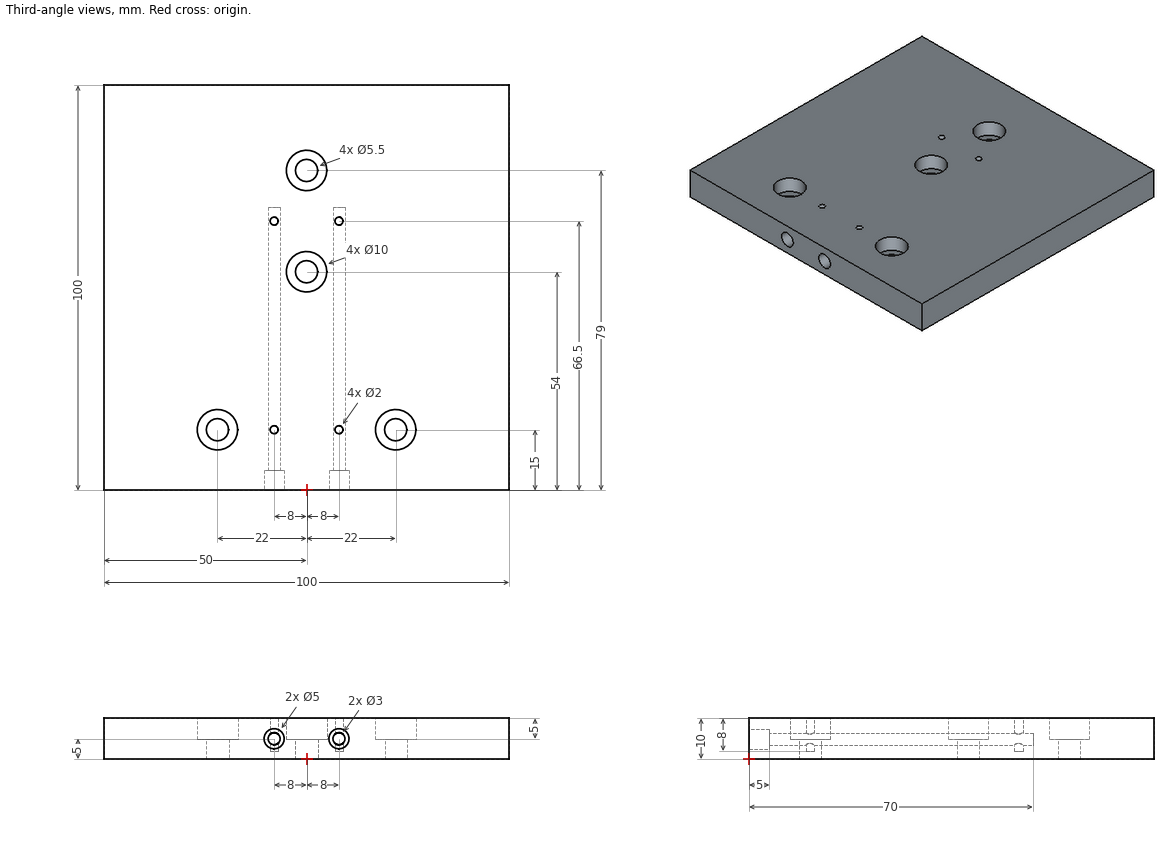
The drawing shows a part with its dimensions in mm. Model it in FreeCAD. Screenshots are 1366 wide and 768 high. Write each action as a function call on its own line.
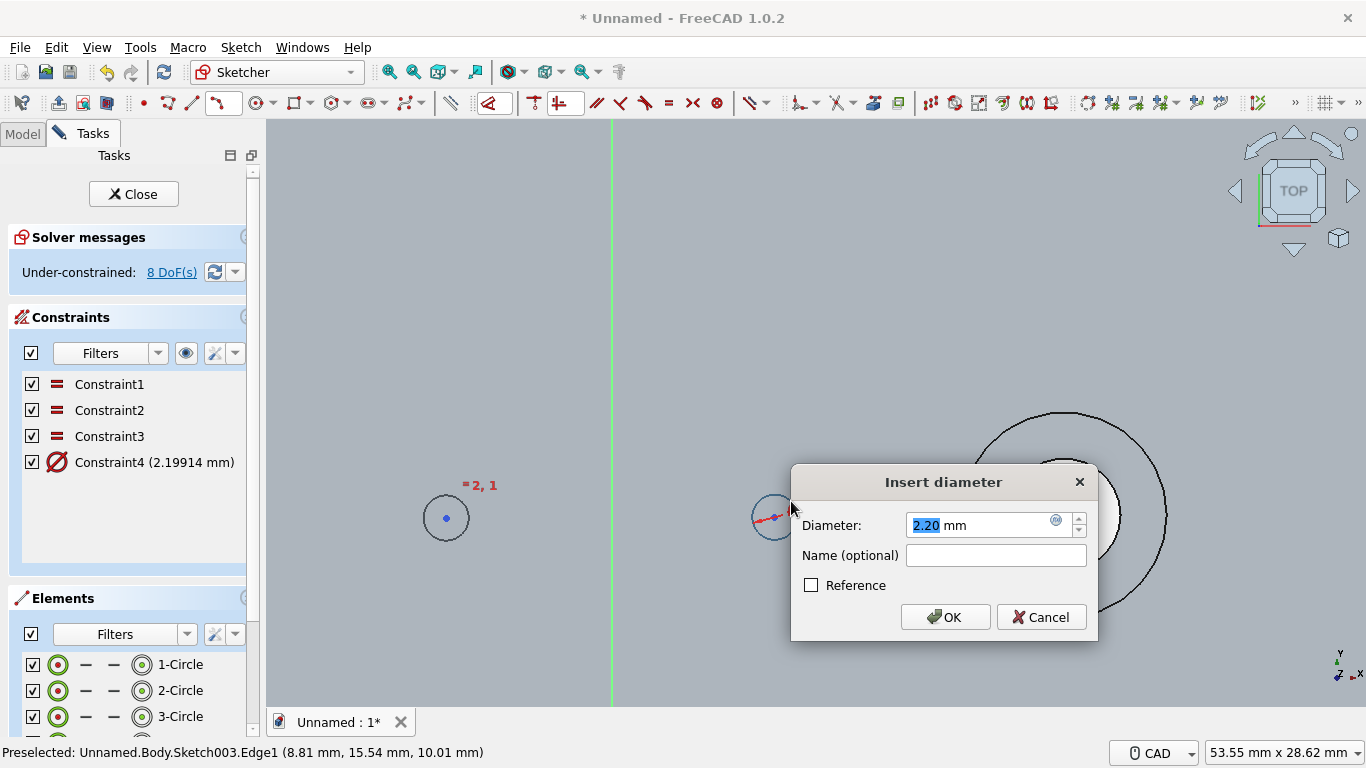
text(2)
key(Return)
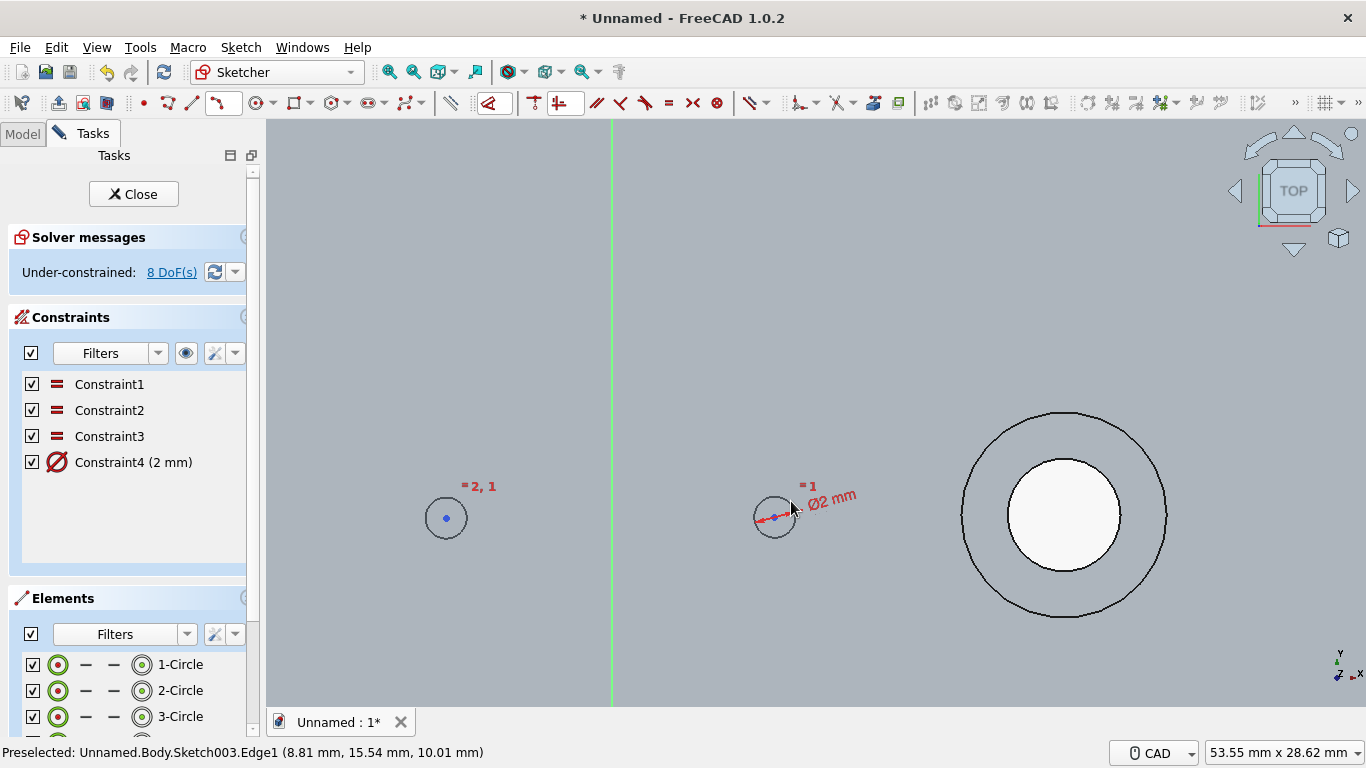
scroll(792, 506, down, 7)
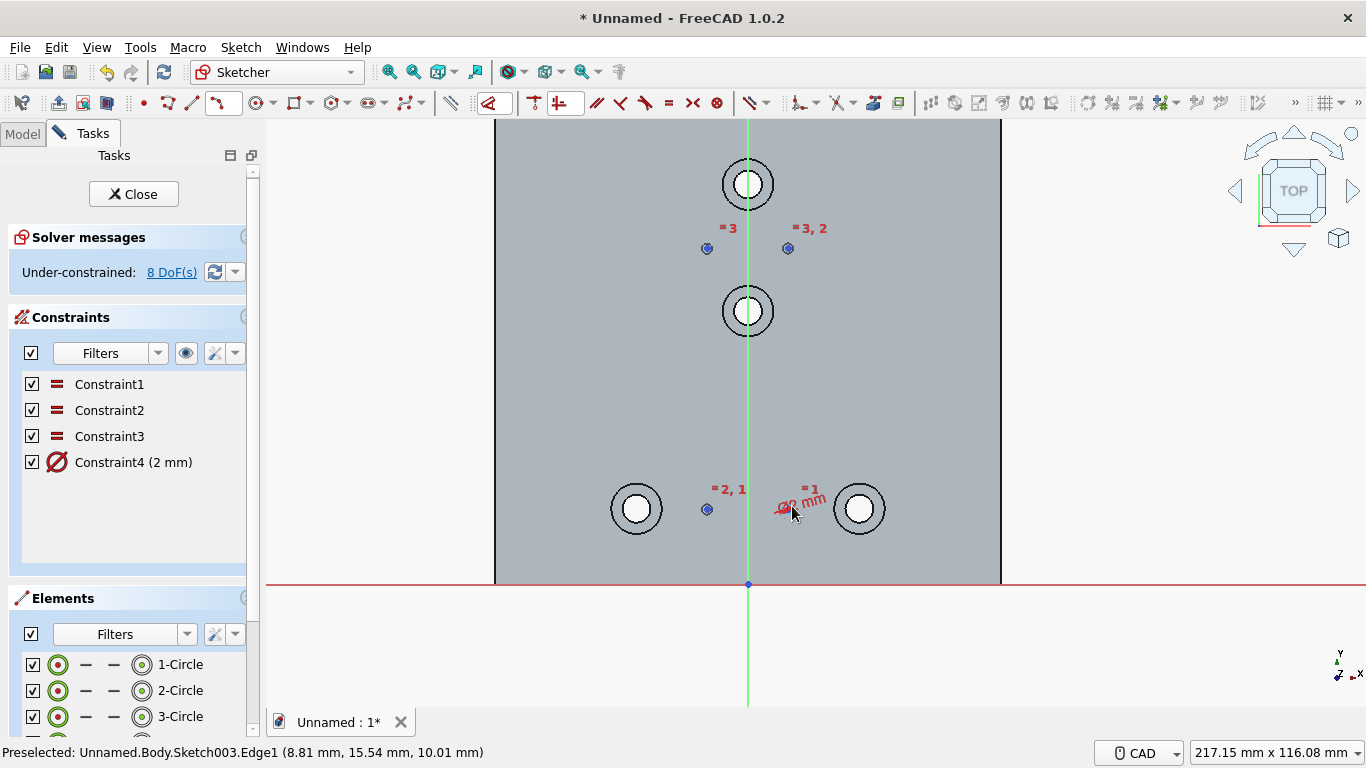
click(788, 509)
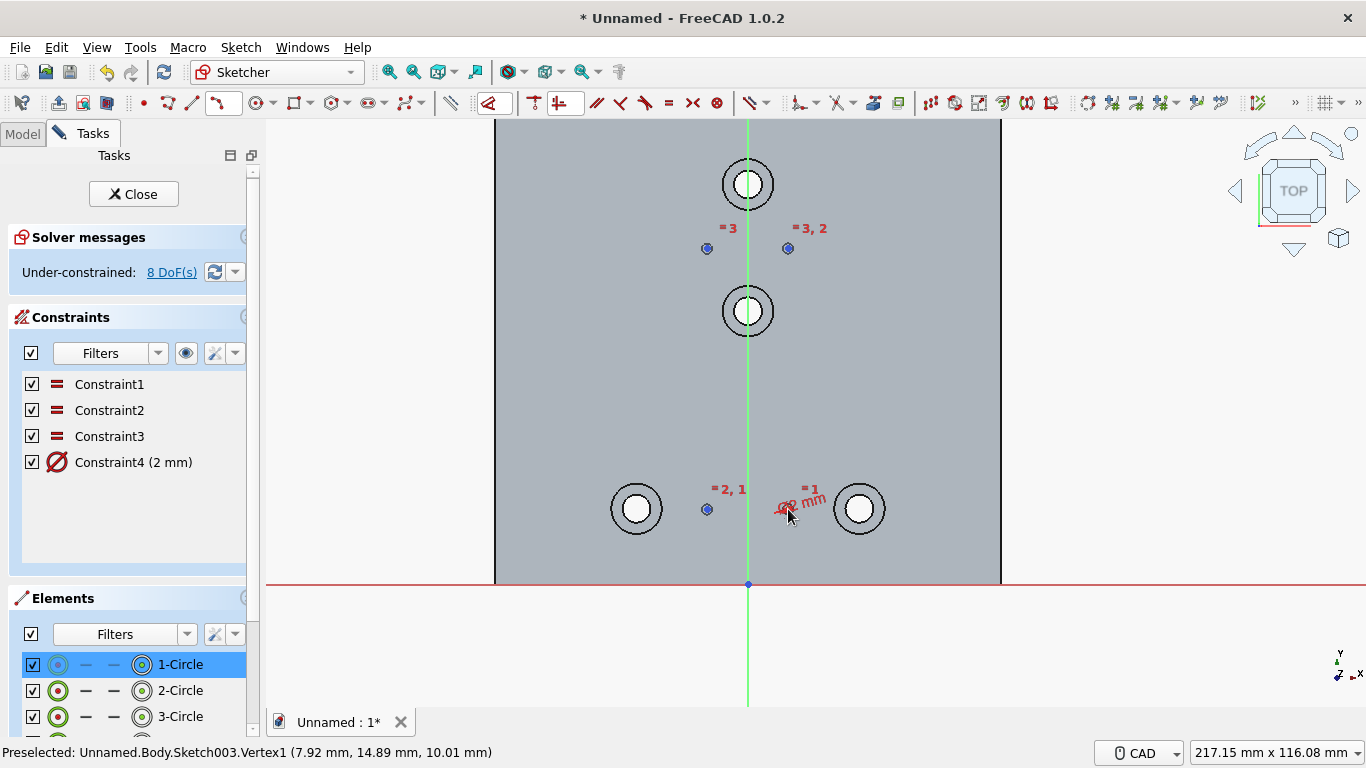
click(506, 104)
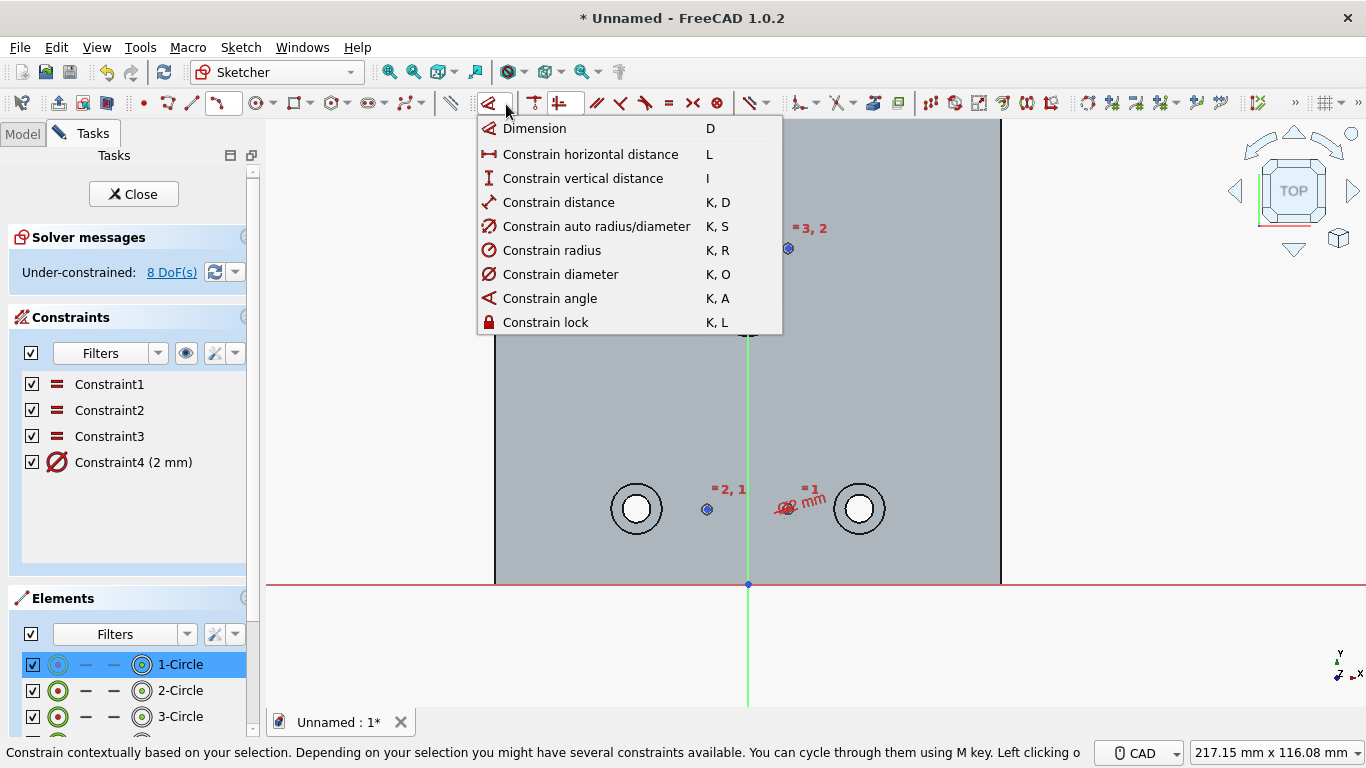
click(630, 154)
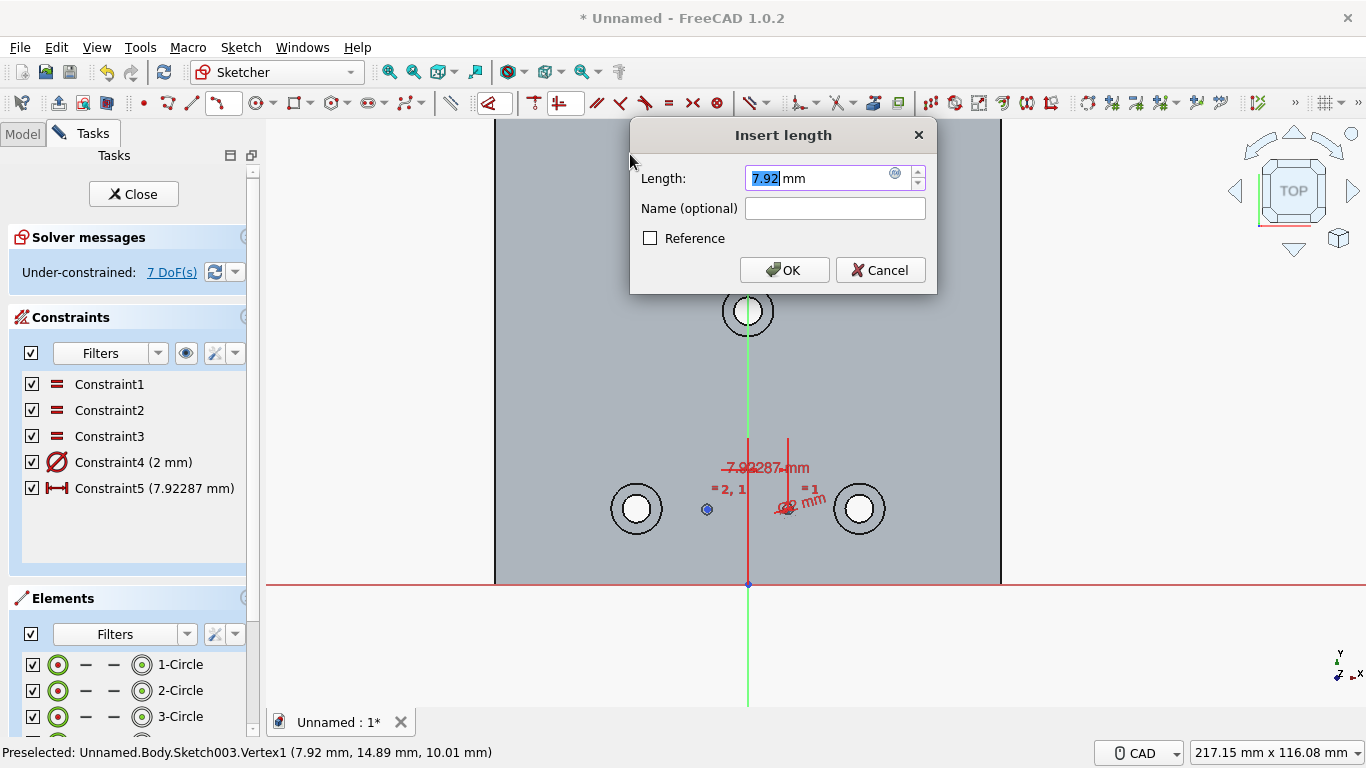
text(8)
key(Return)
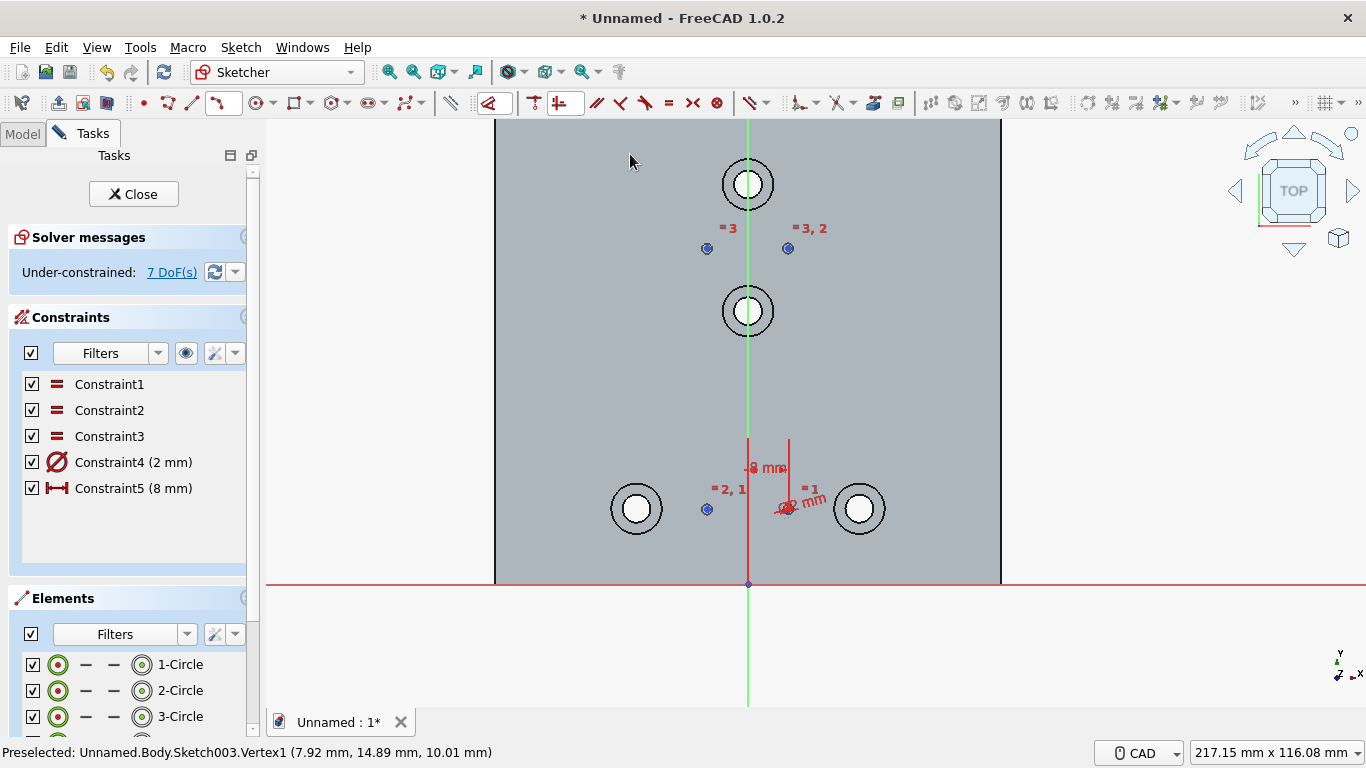
click(707, 509)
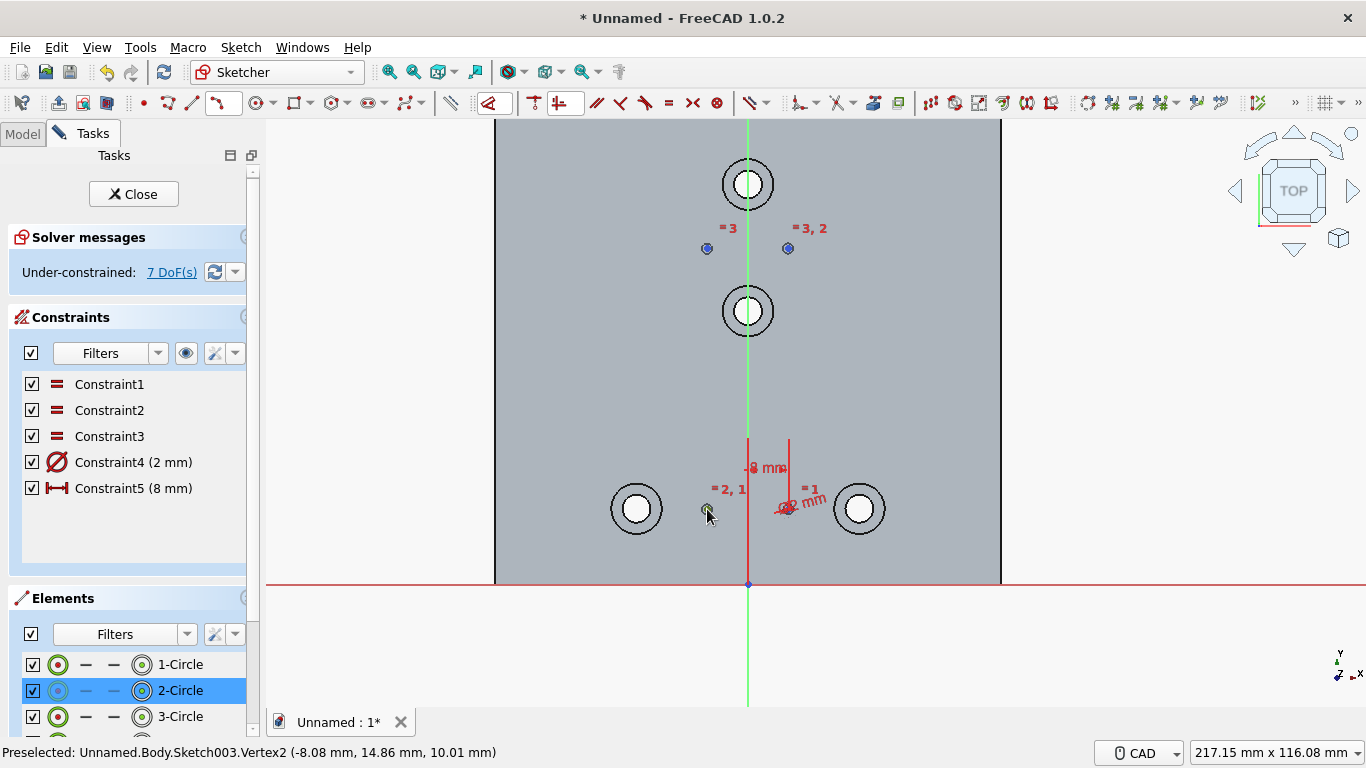
click(506, 104)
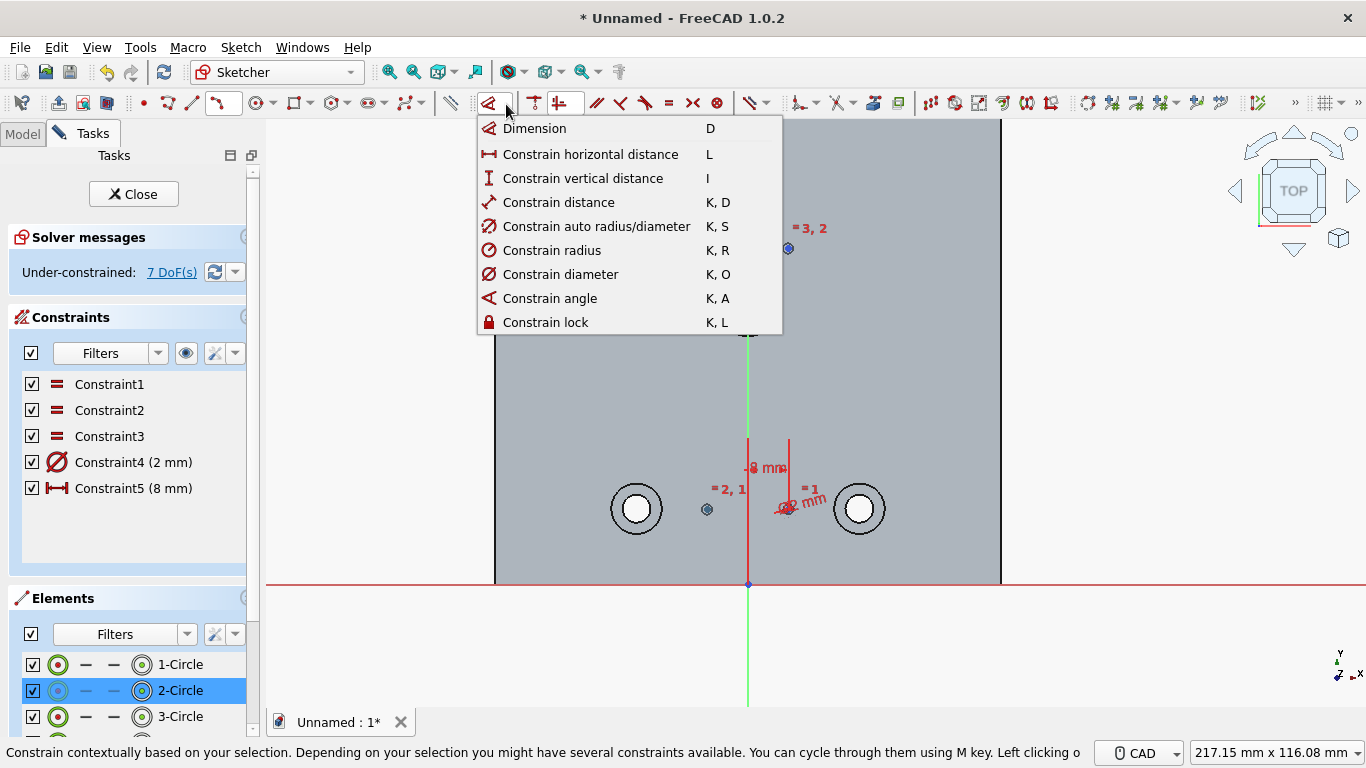
click(630, 154)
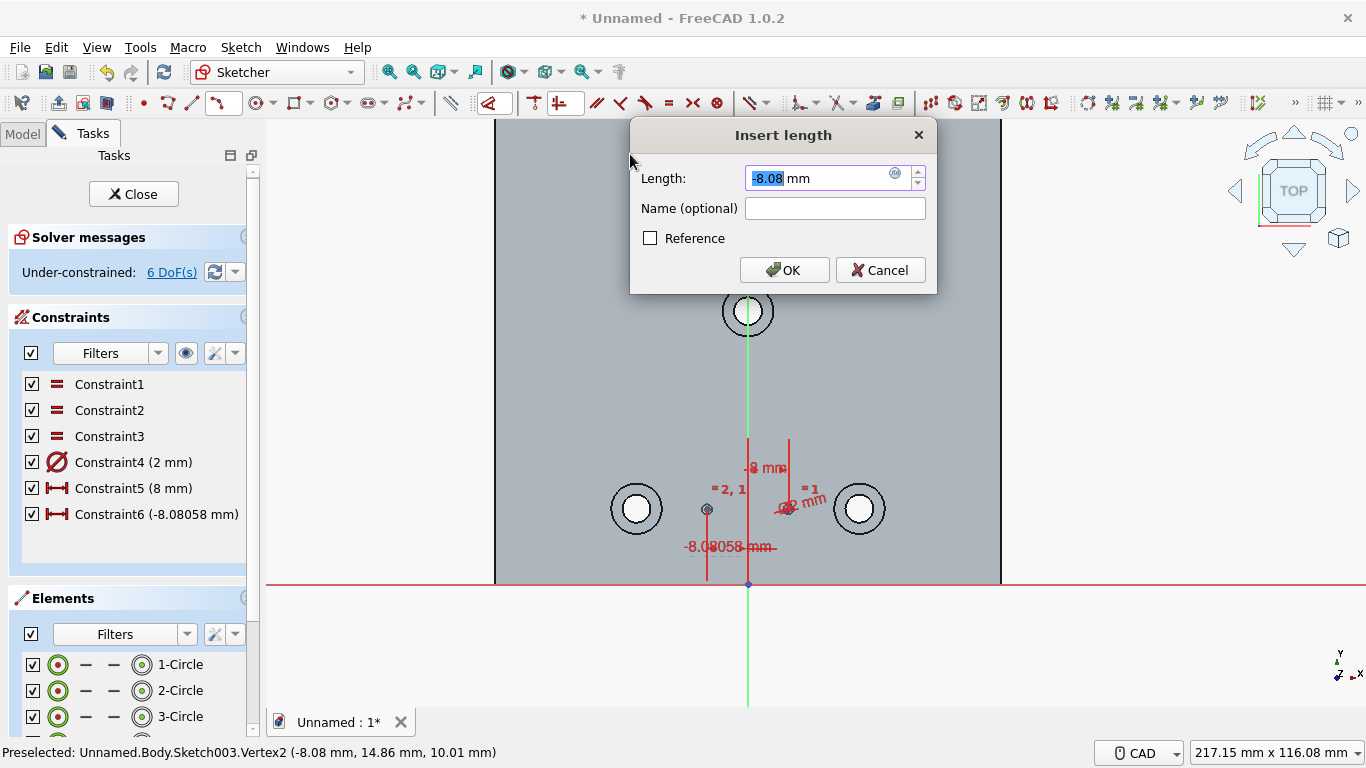
text(-8)
key(Return)